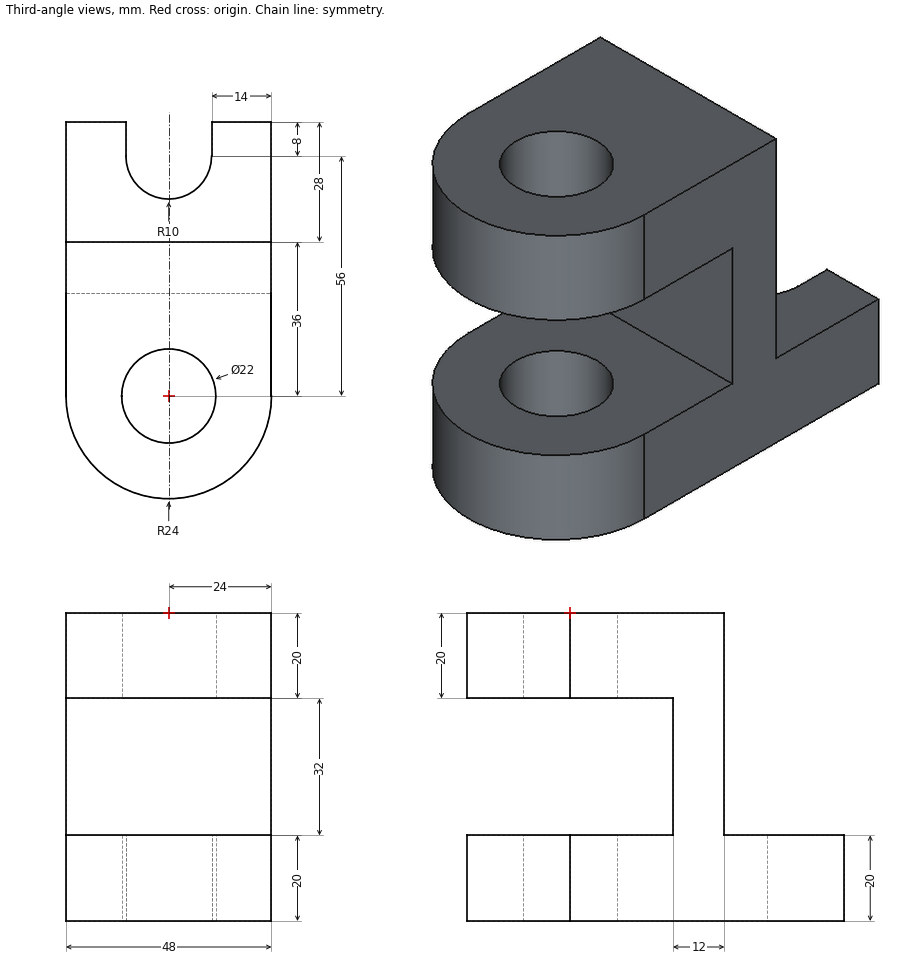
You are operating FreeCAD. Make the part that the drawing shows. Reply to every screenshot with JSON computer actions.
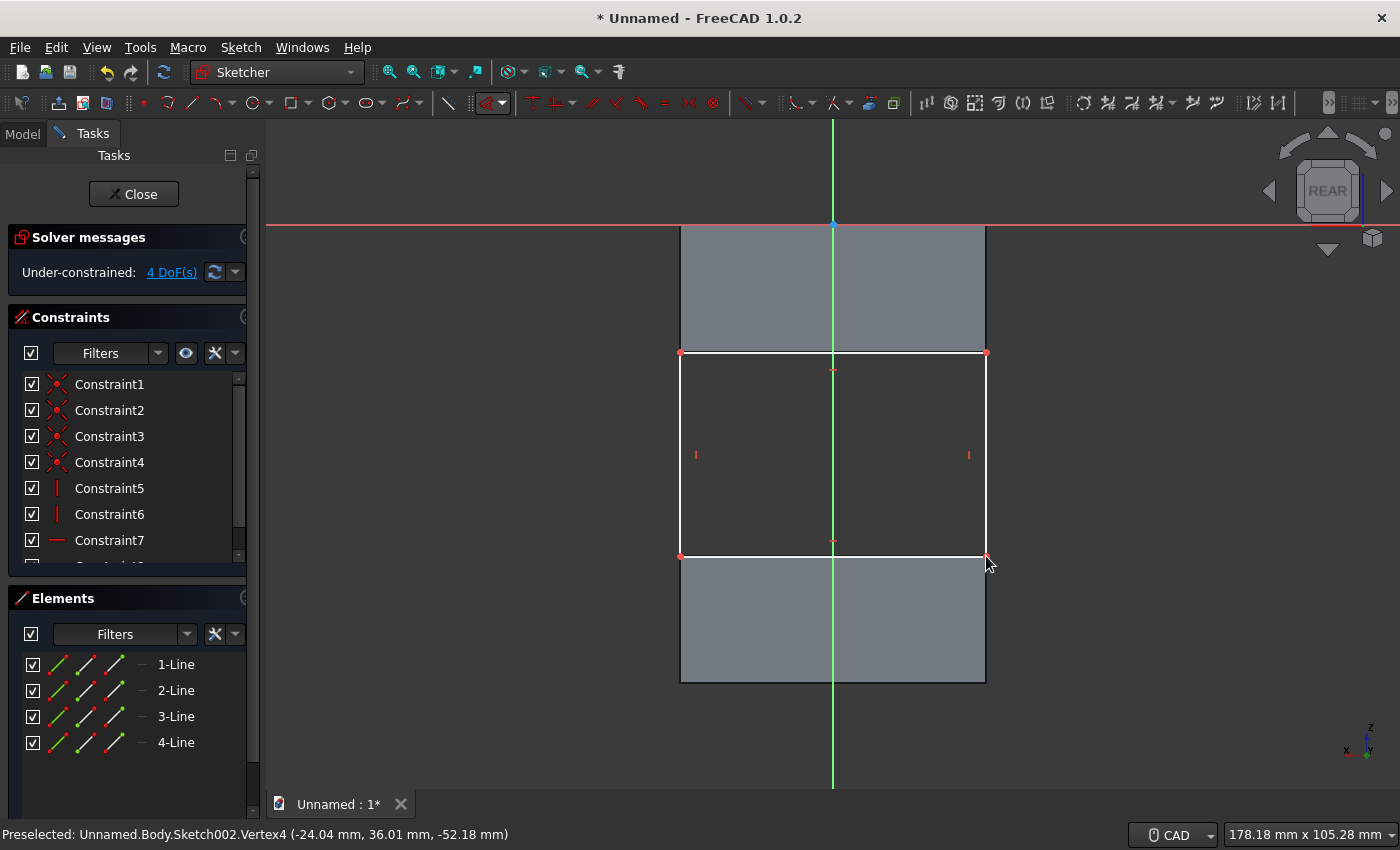
{"action": "left_click", "coordinate": [680, 414]}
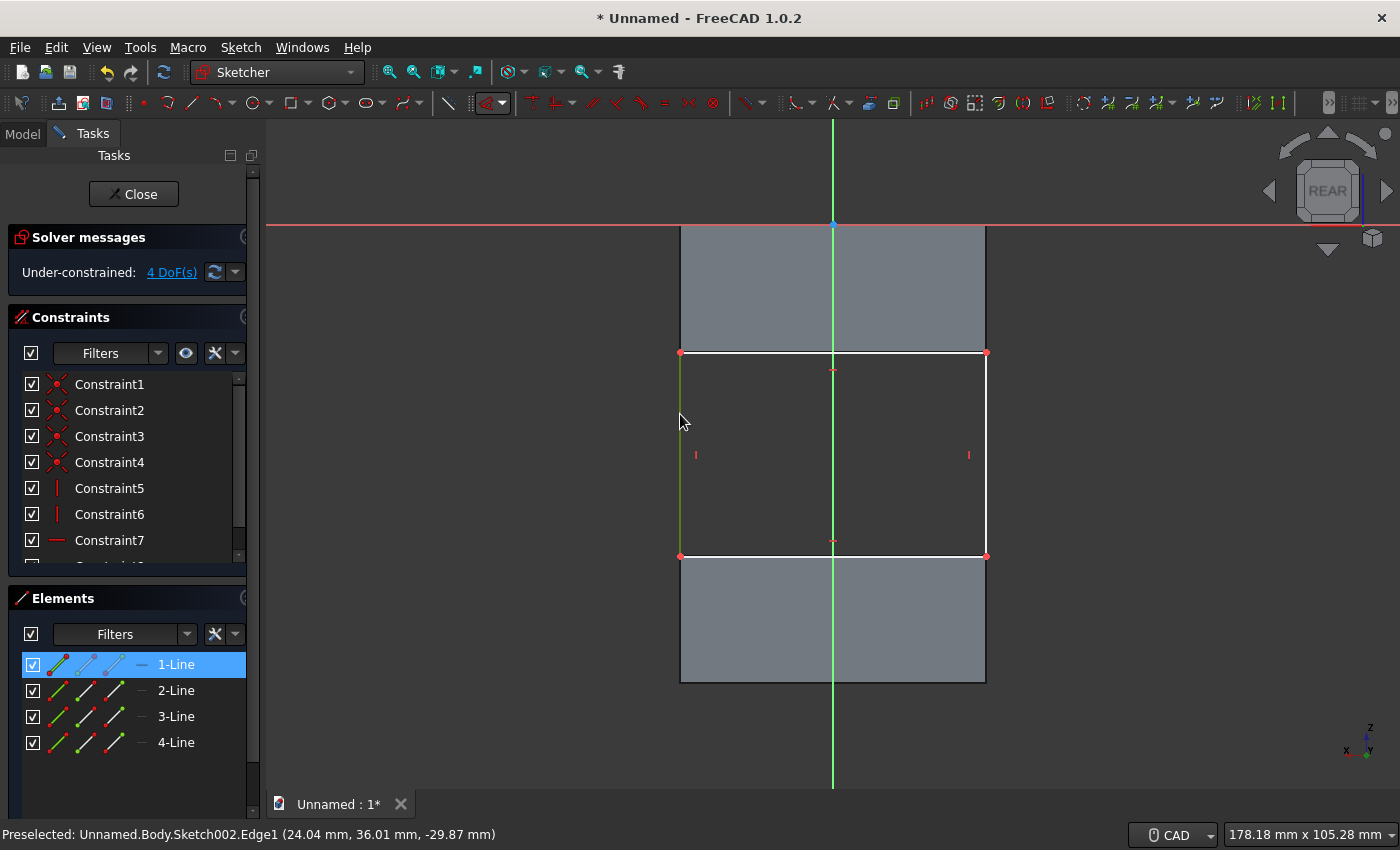
{"action": "left_click", "coordinate": [504, 104]}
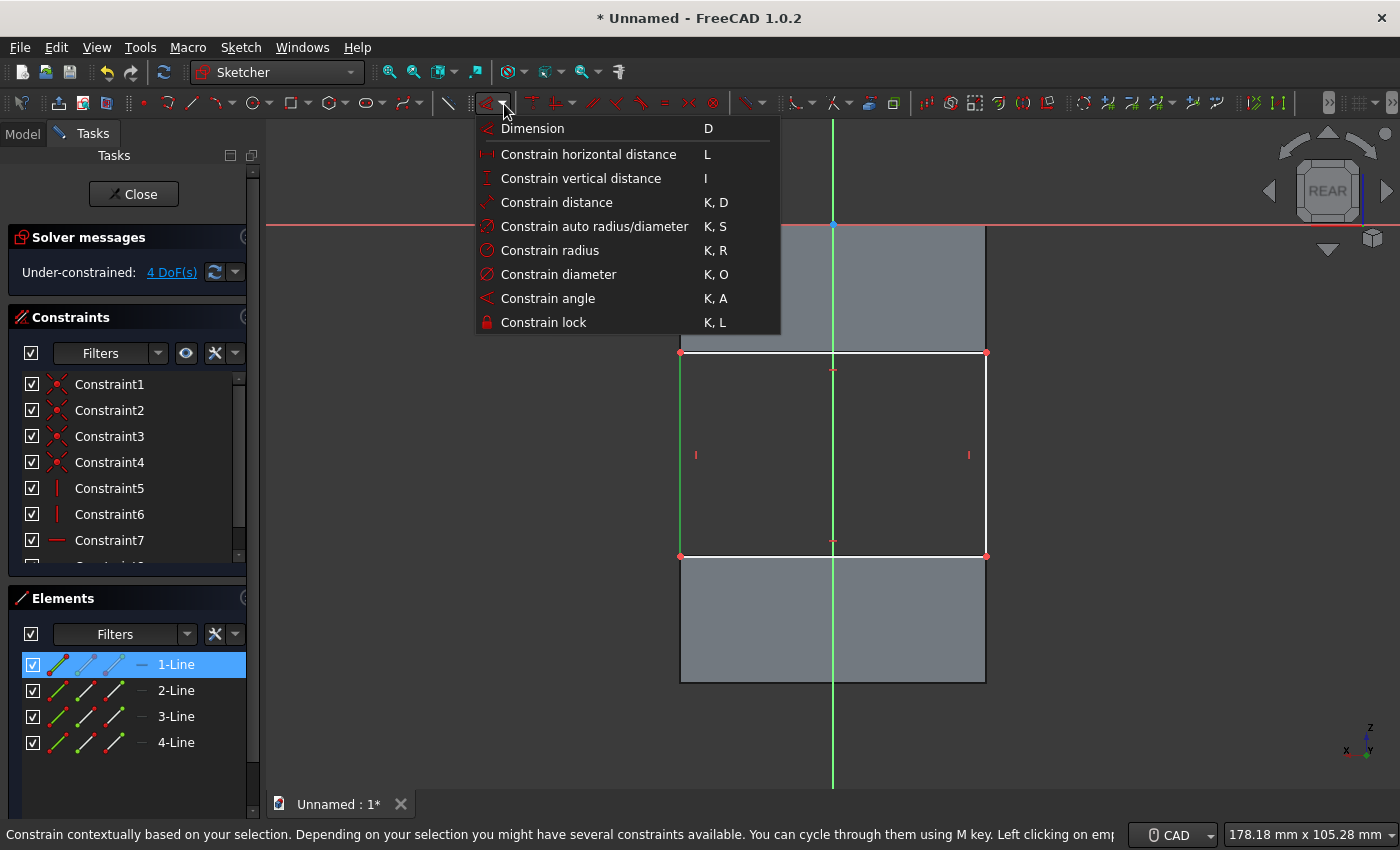
{"action": "left_click", "coordinate": [628, 178]}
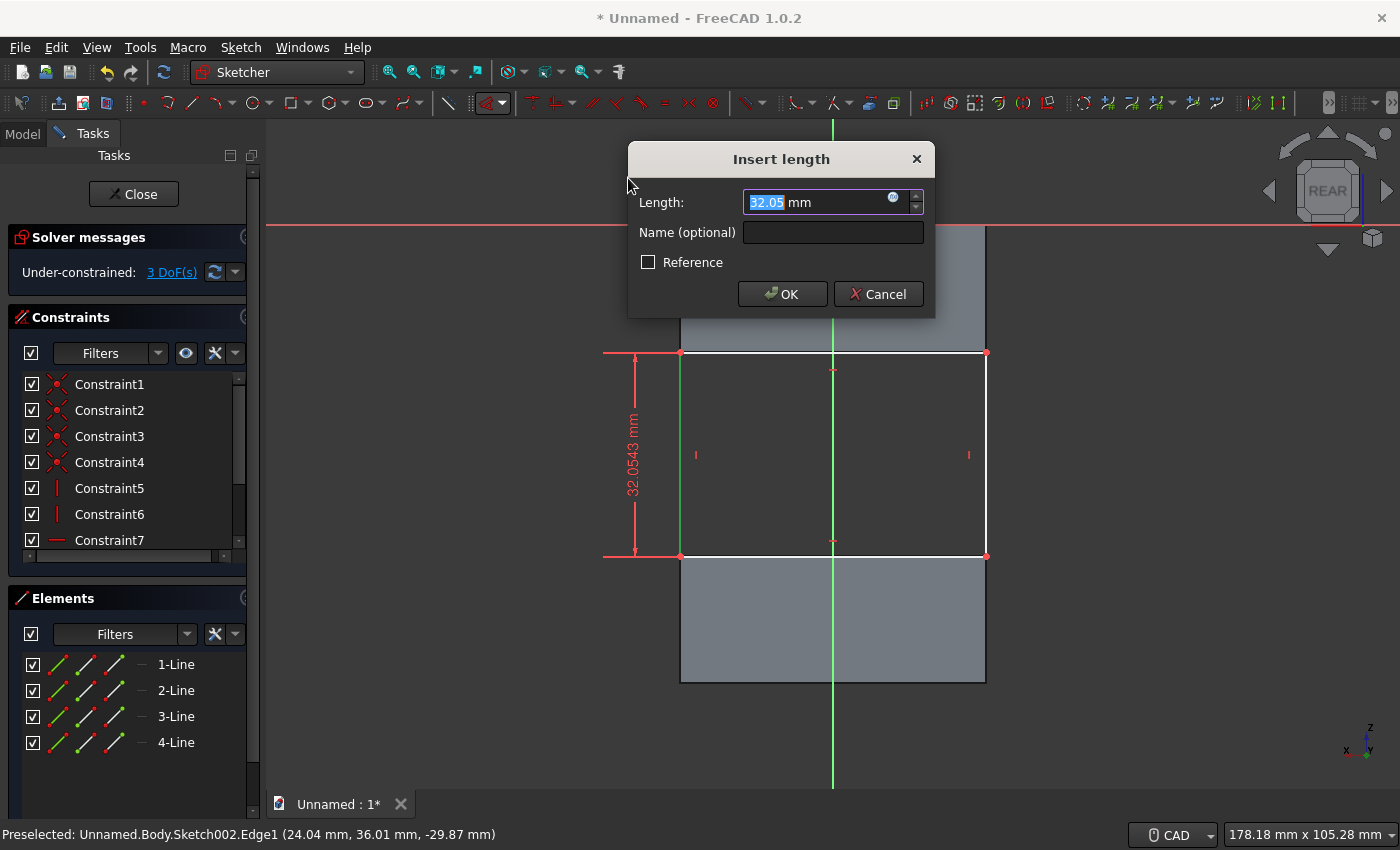
{"action": "type", "text": "32"}
{"action": "key", "text": "Return"}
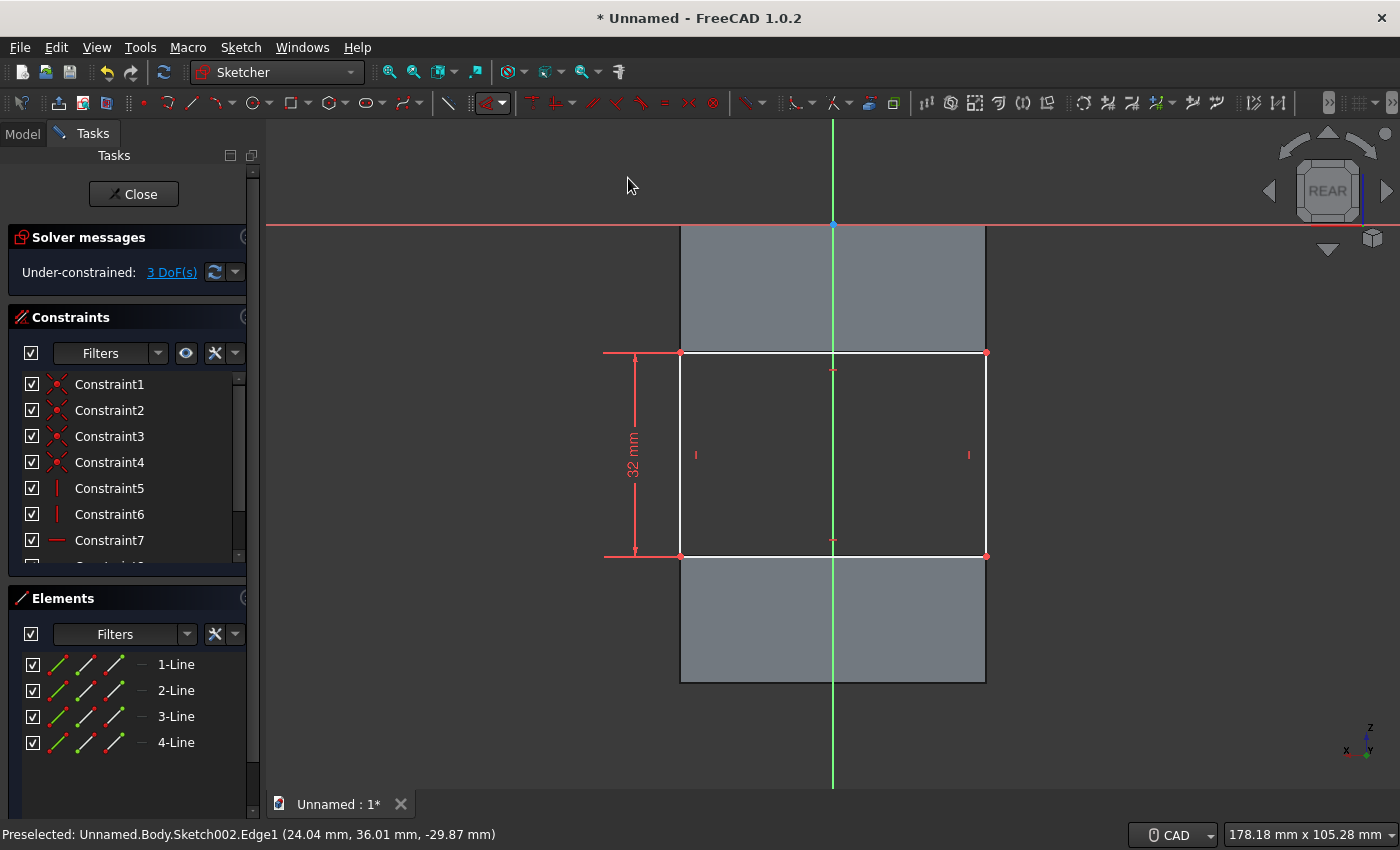
{"action": "left_click", "coordinate": [772, 557]}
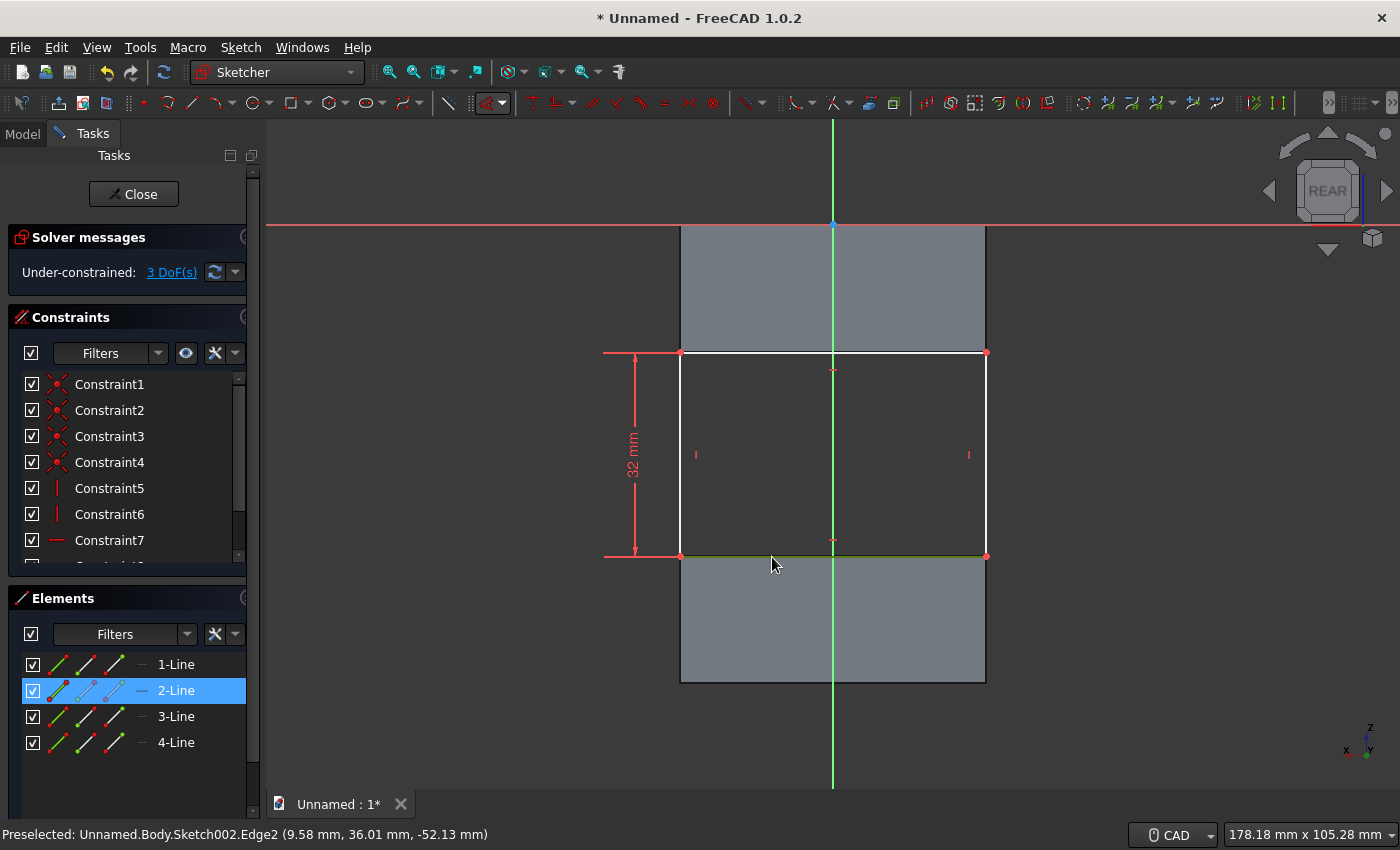
{"action": "key", "text": "l"}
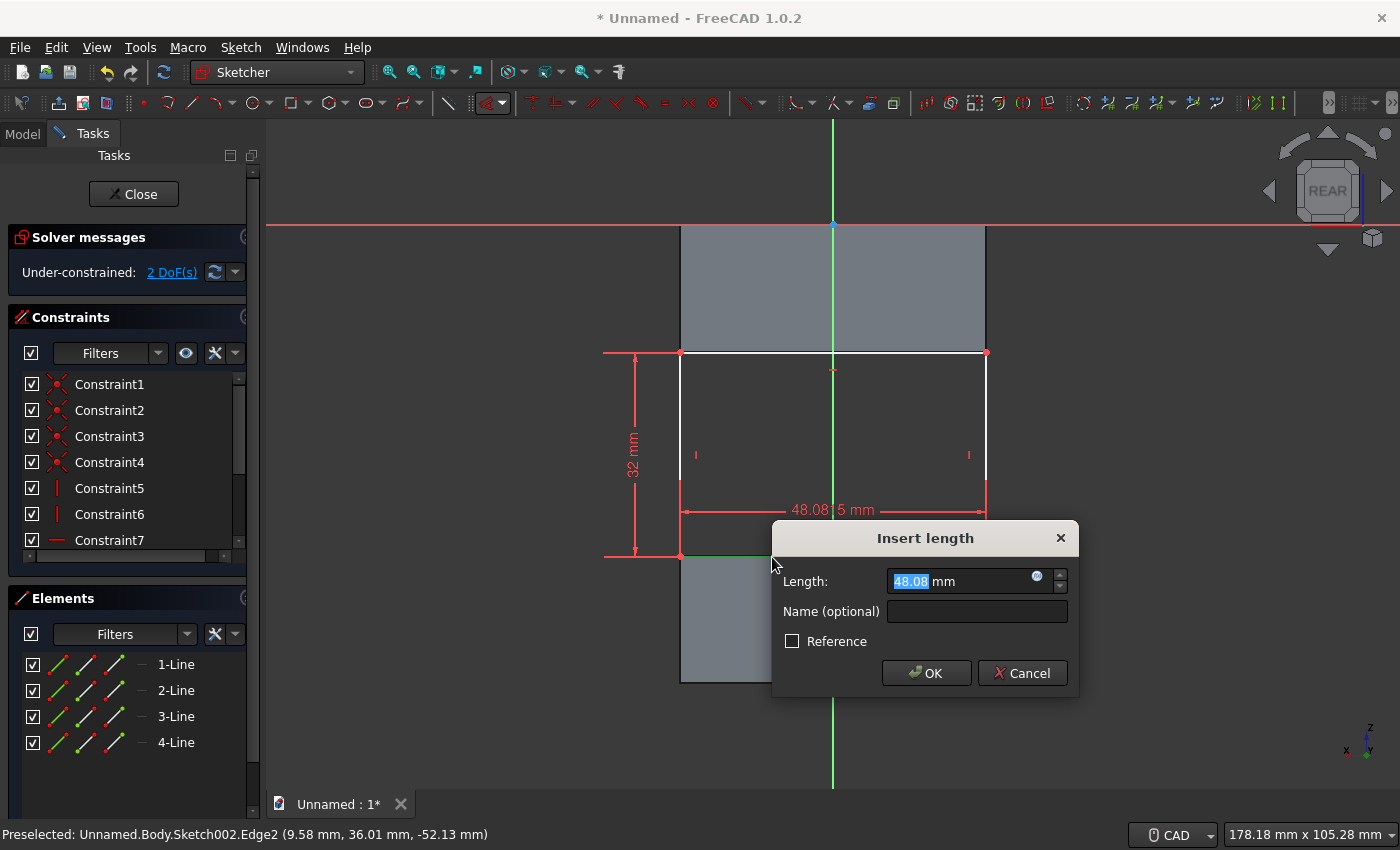
{"action": "type", "text": "48"}
{"action": "key", "text": "Return"}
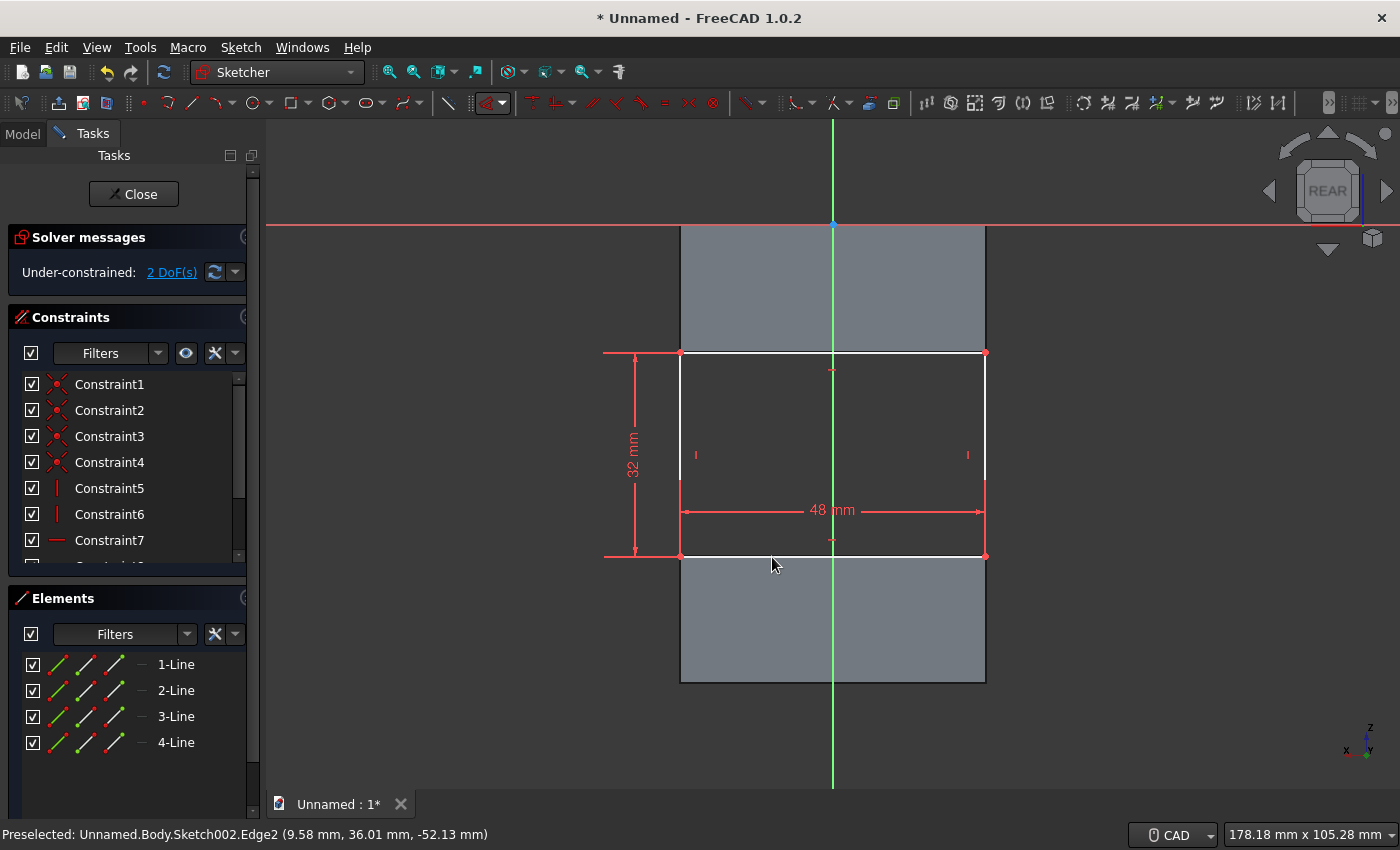
{"action": "left_click", "coordinate": [680, 353]}